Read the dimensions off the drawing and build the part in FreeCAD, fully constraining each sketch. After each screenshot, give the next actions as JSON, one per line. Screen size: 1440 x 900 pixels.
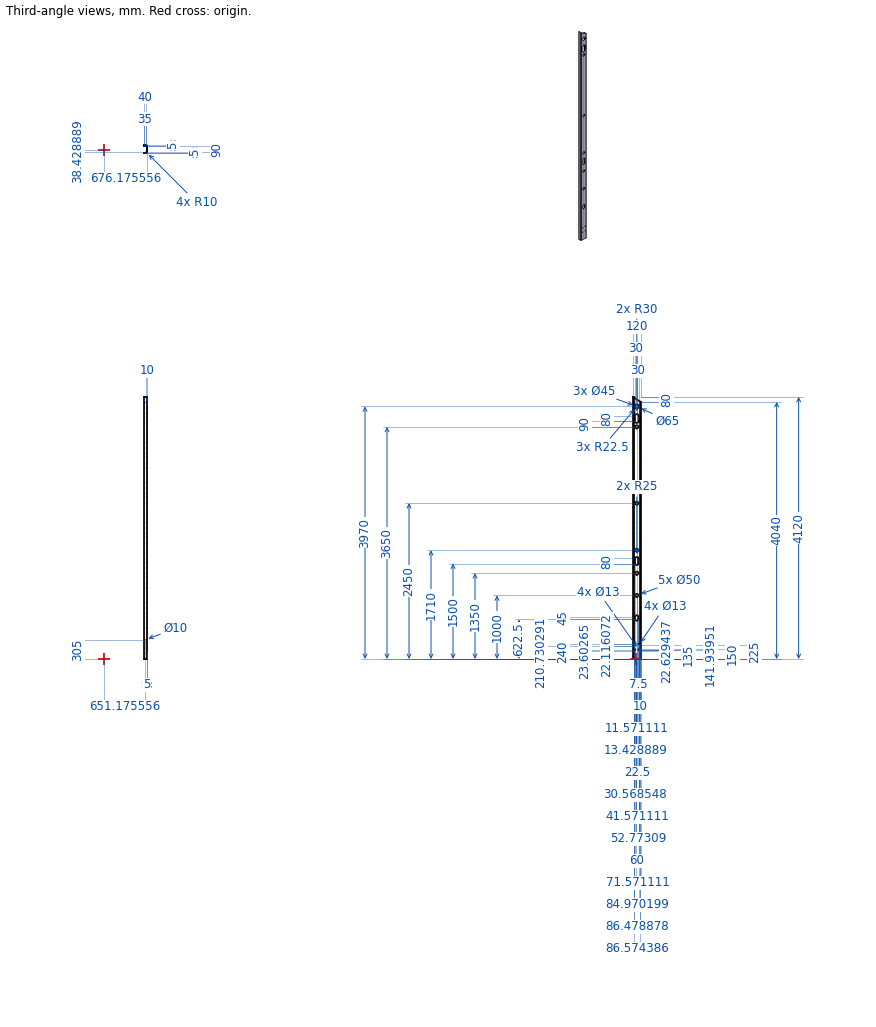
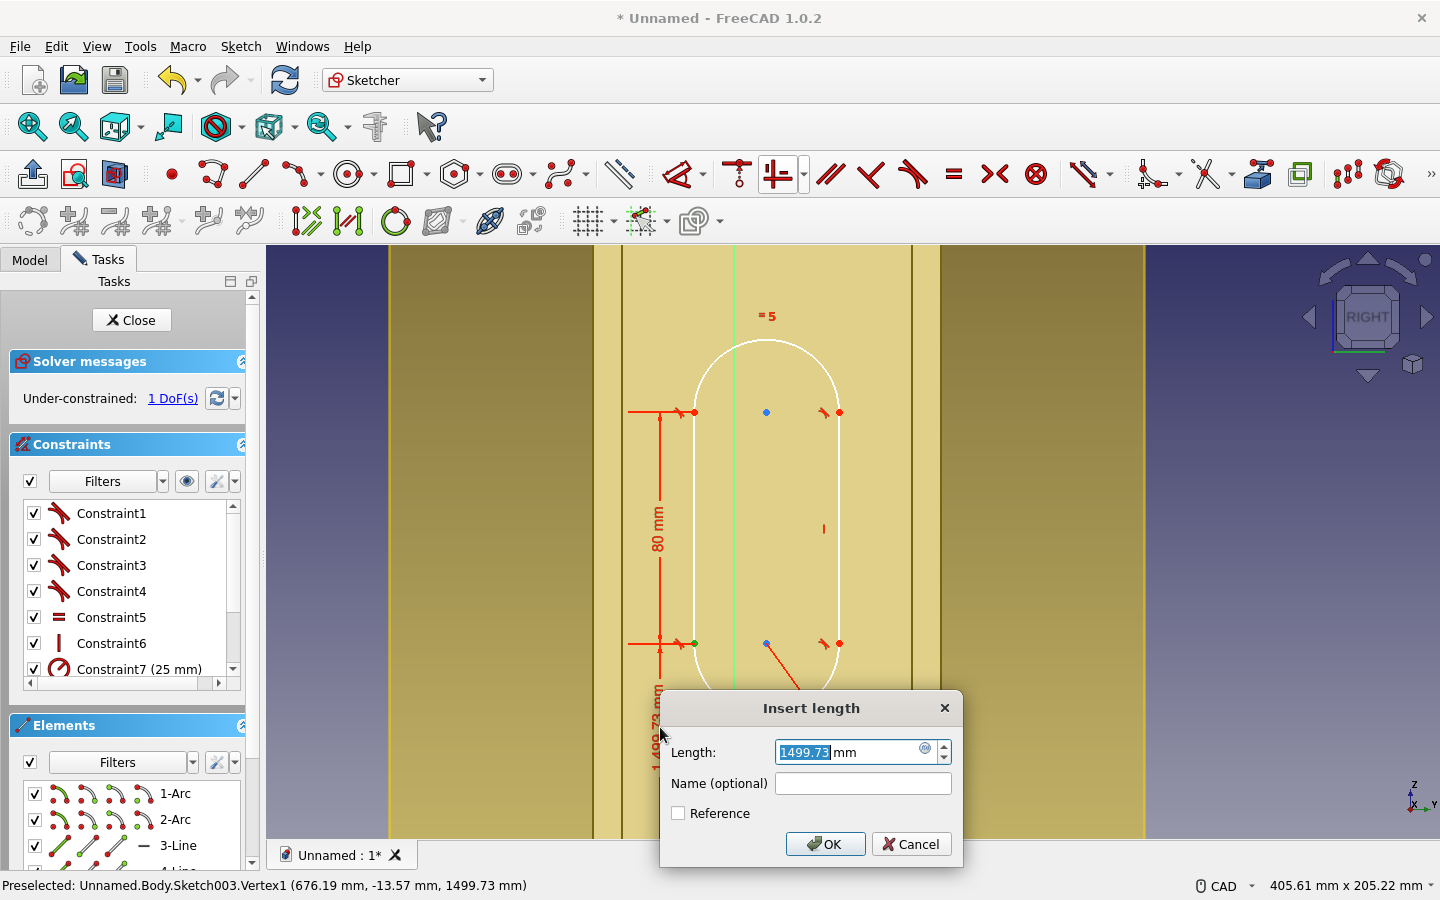
{"action": "type", "text": "1500"}
{"action": "key", "text": "Return"}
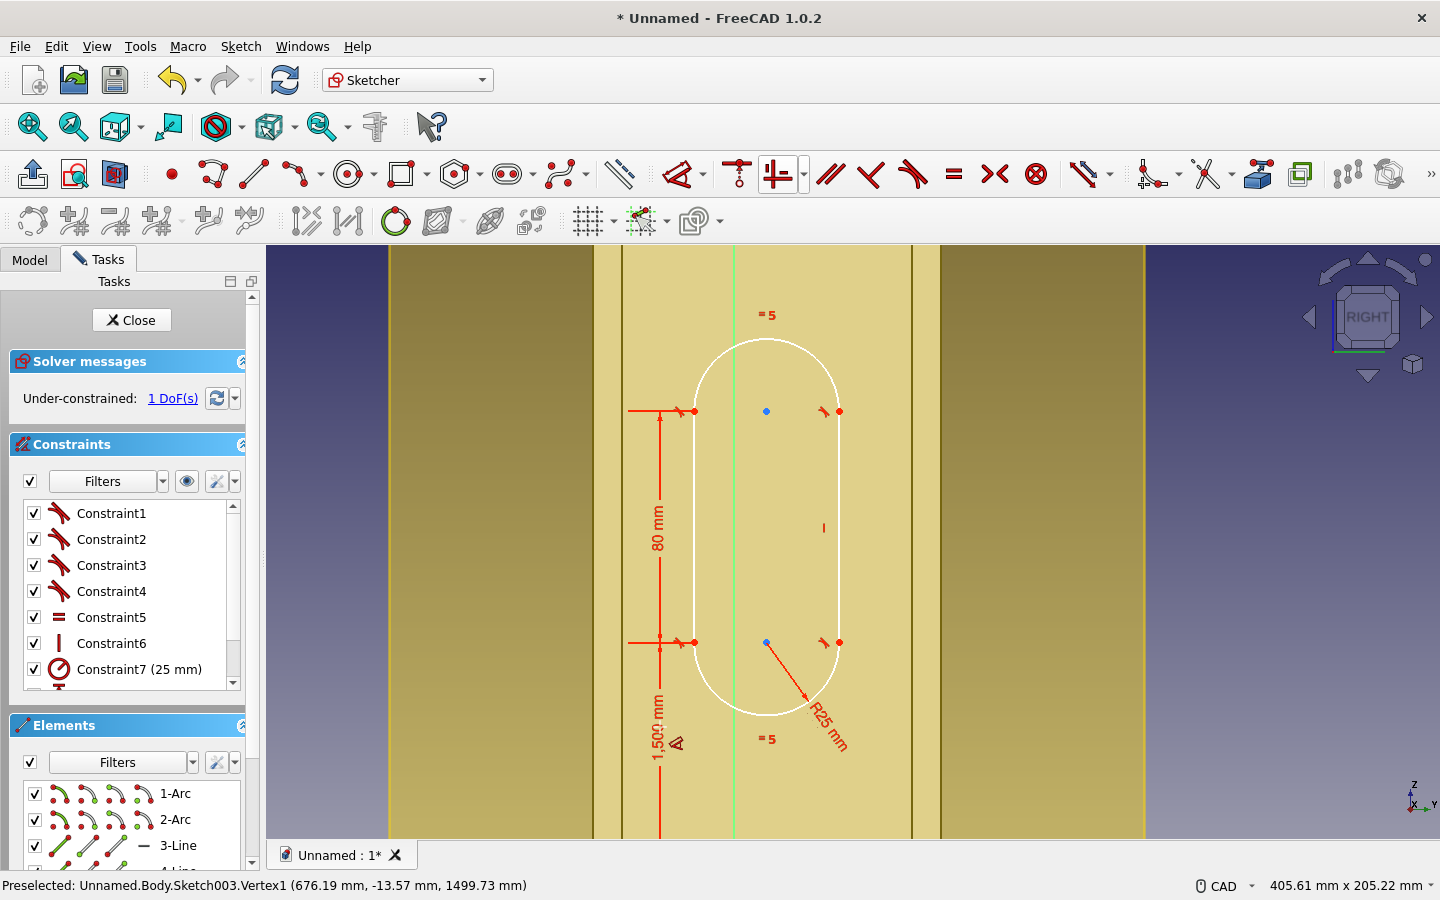
{"action": "left_click", "coordinate": [694, 643]}
{"action": "left_click", "coordinate": [714, 609]}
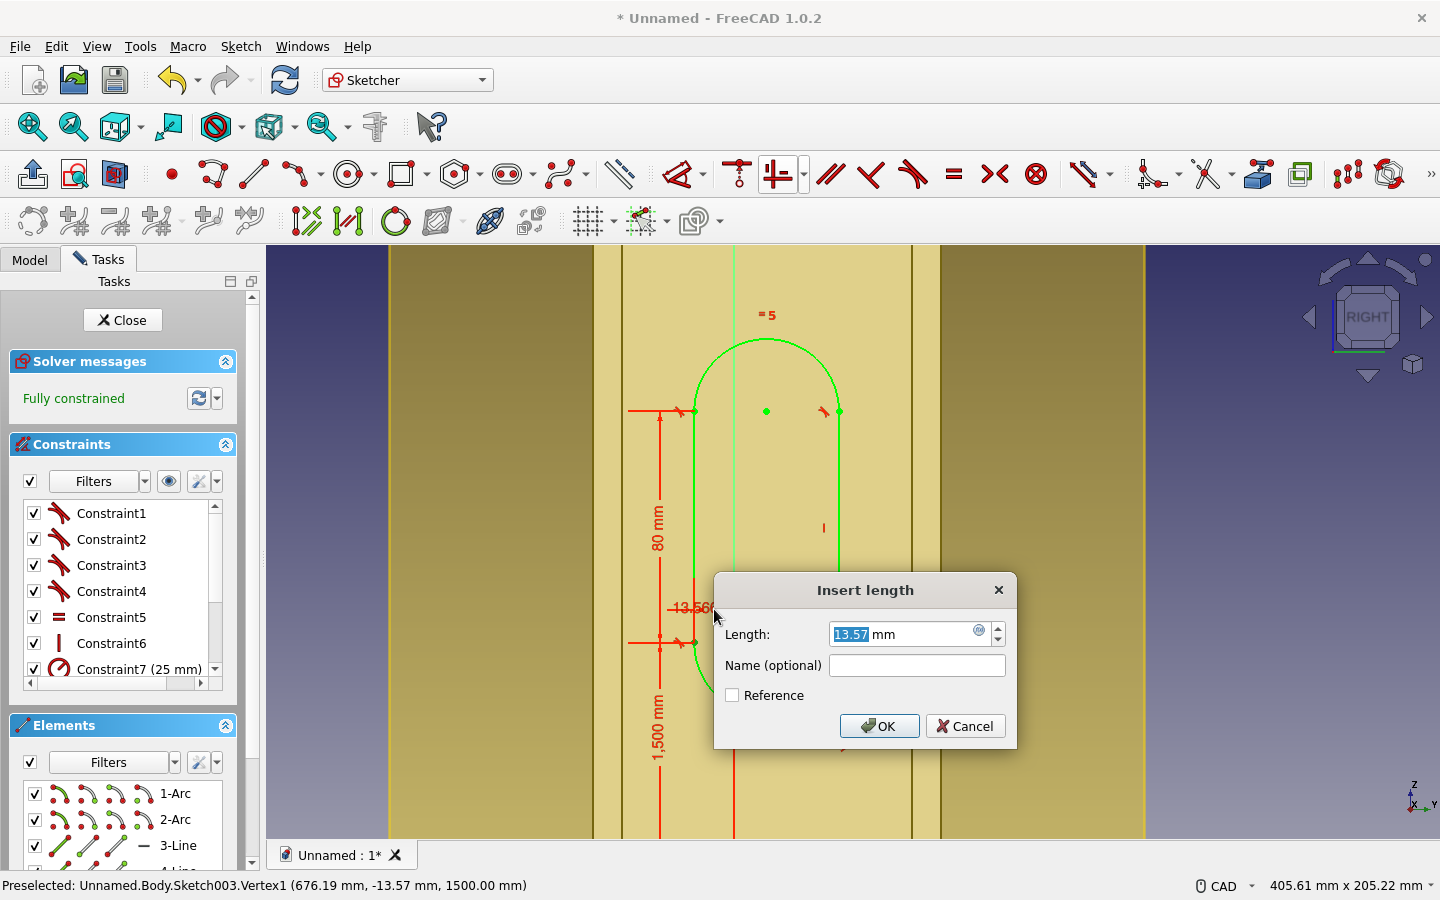
{"action": "type", "text": "13.428889"}
{"action": "key", "text": "Return"}
{"action": "key", "text": "Escape"}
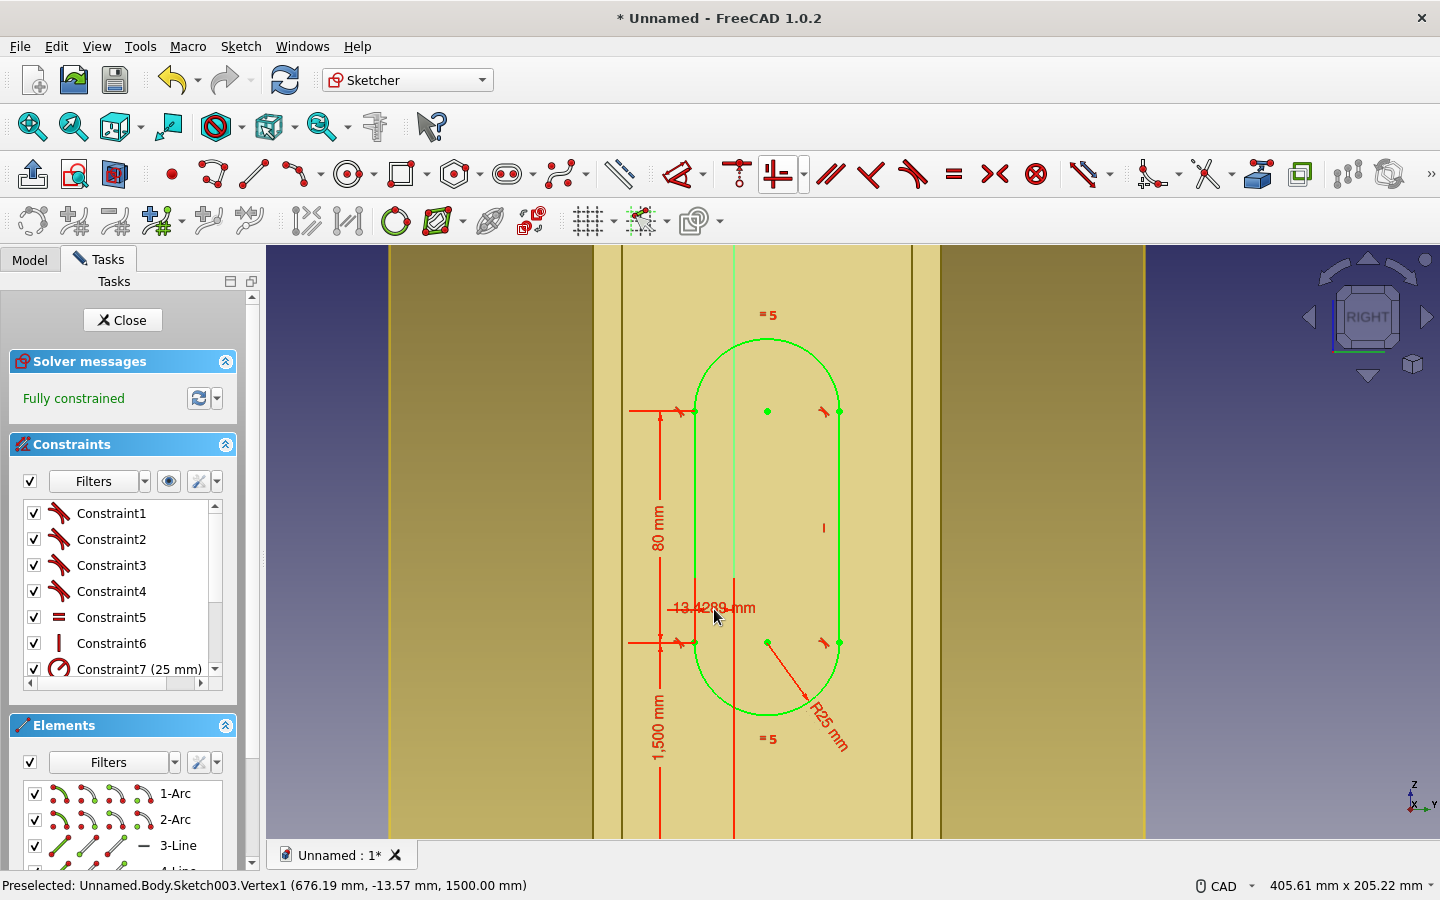
{"action": "left_click", "coordinate": [123, 320]}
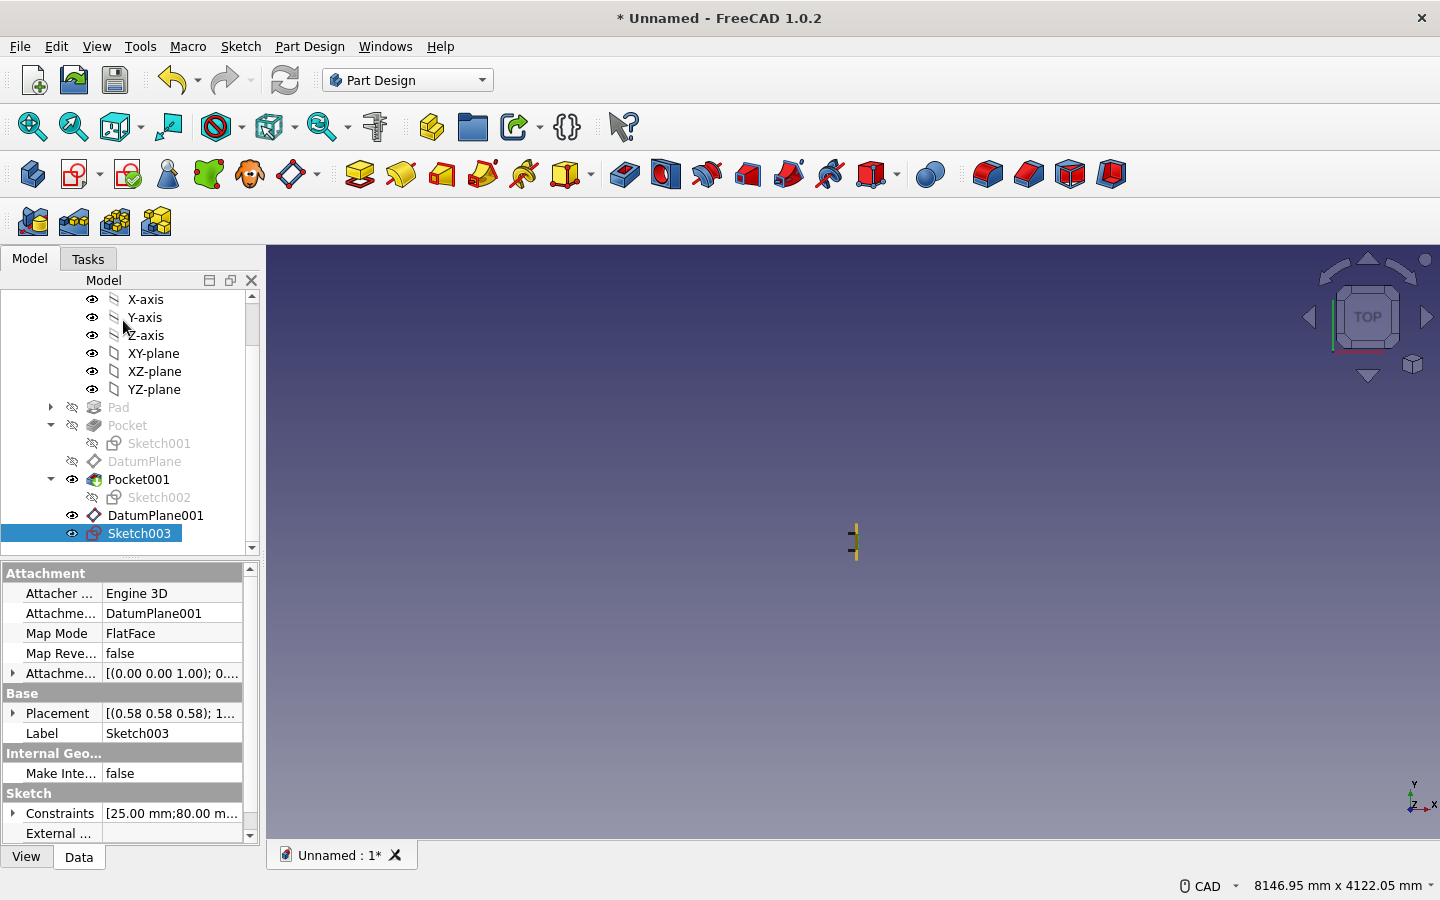
{"action": "left_click", "coordinate": [625, 174]}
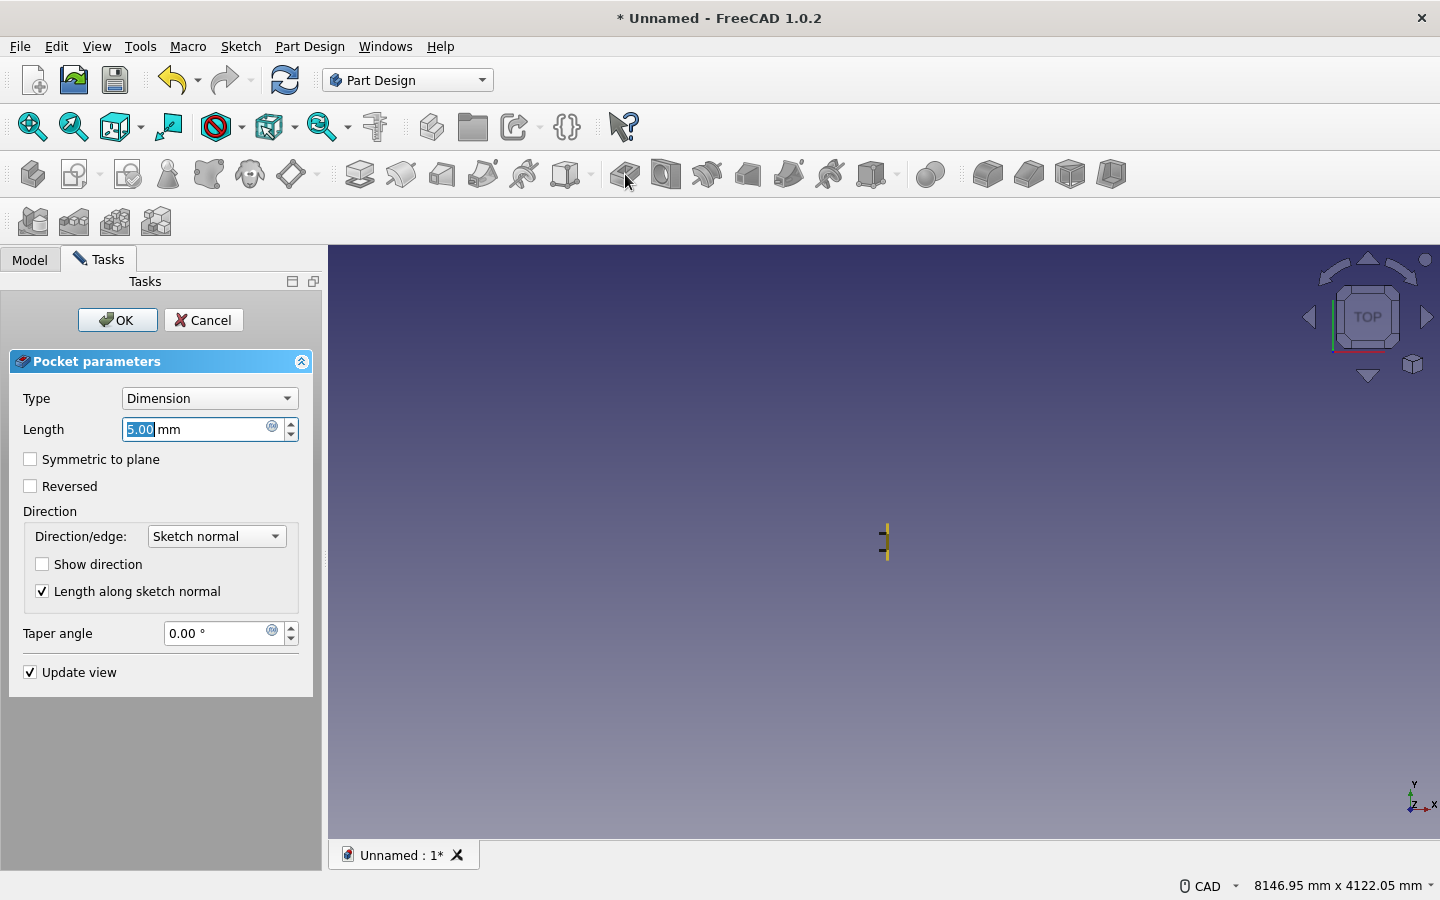
{"action": "type", "text": "10"}
{"action": "key", "text": "Tab"}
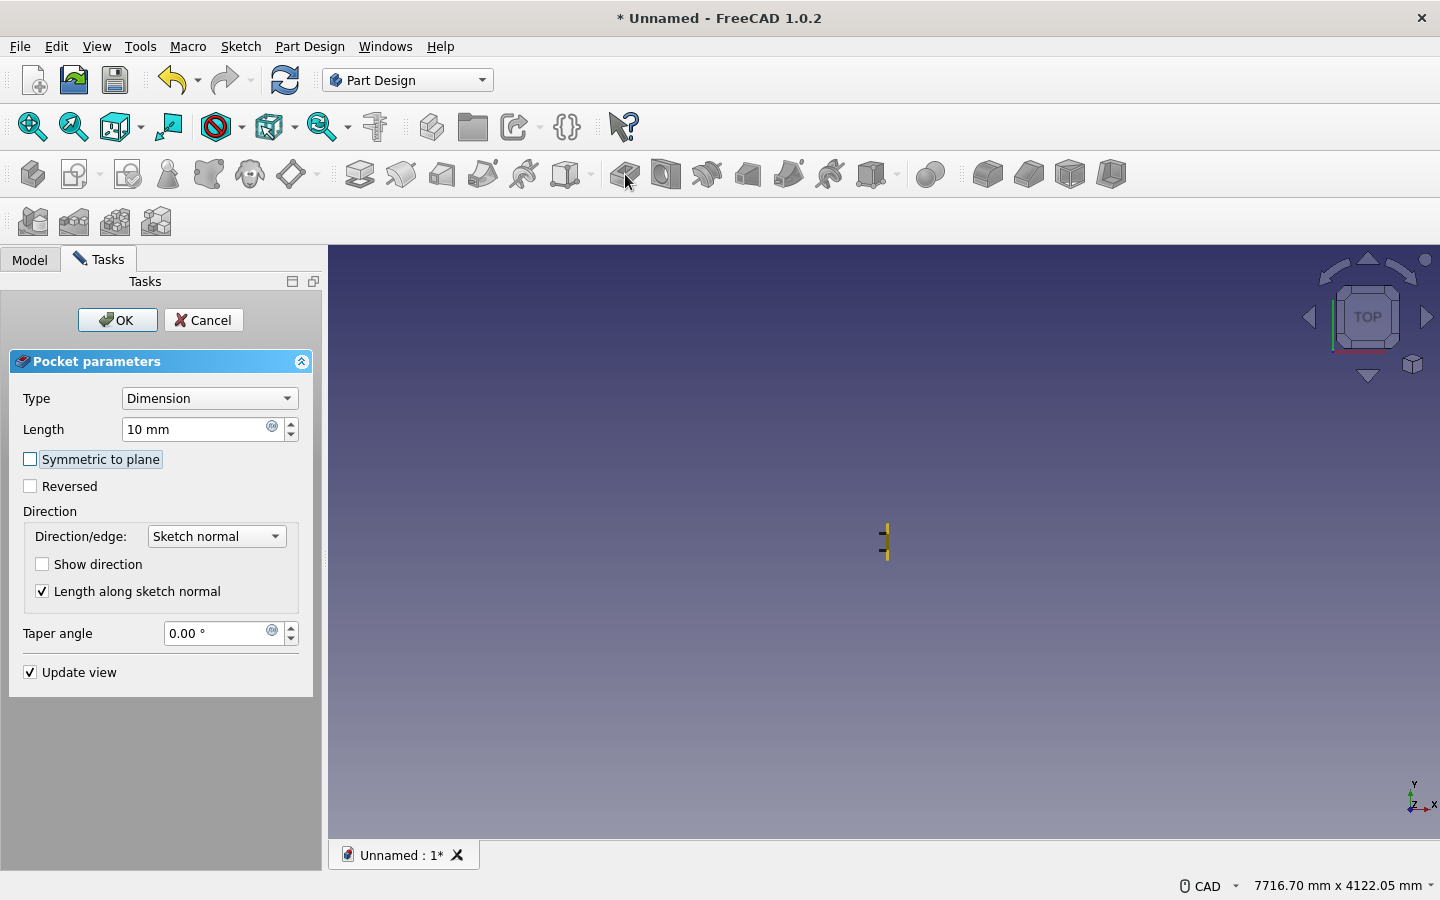
{"action": "left_click", "coordinate": [118, 320]}